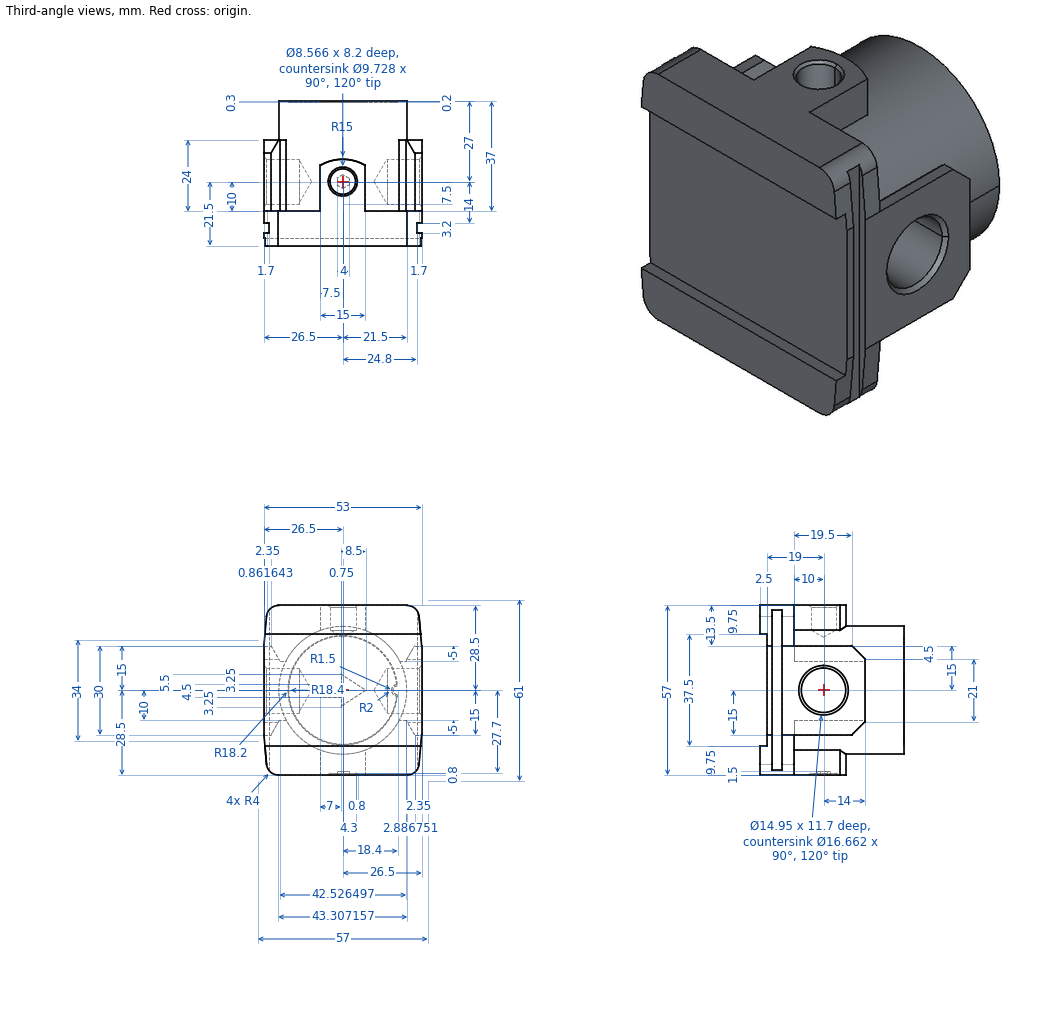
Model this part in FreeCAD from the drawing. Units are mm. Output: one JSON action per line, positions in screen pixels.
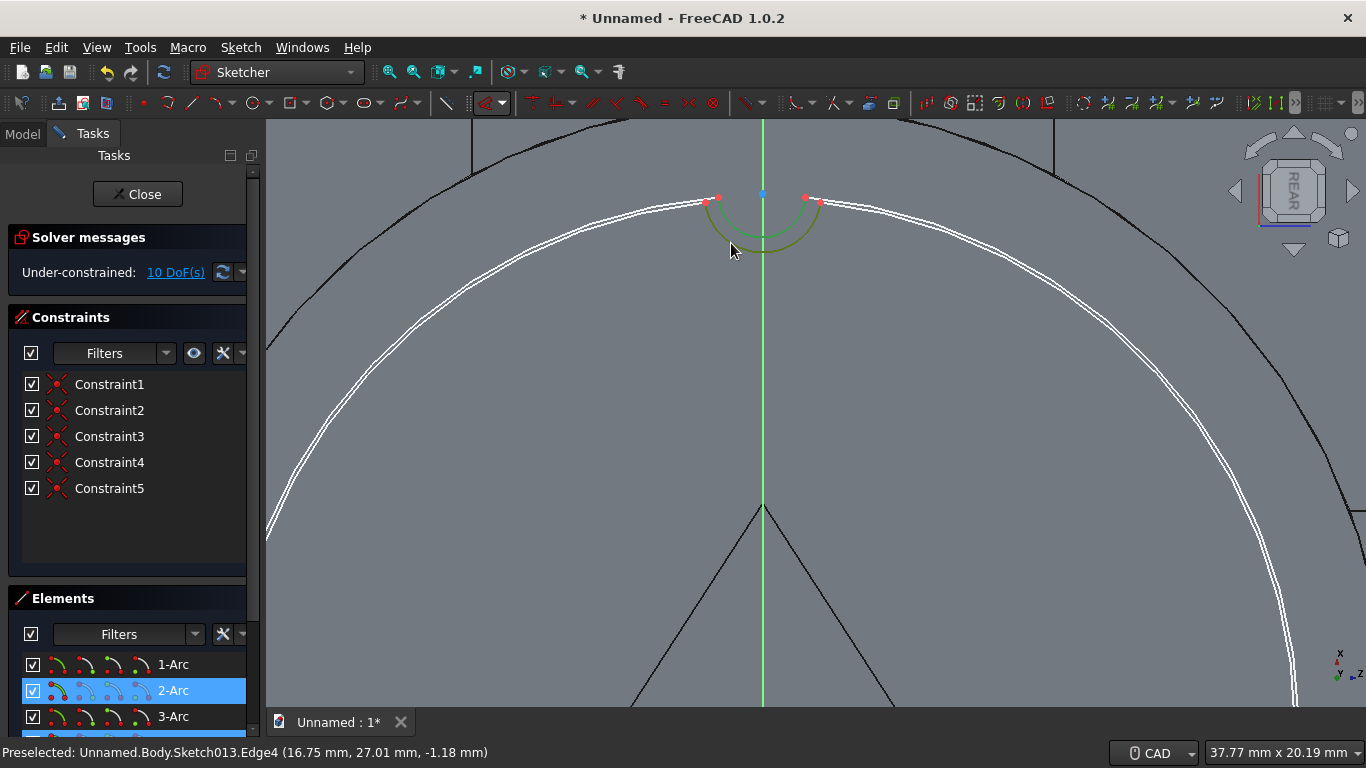
{"action": "left_click", "coordinate": [532, 104]}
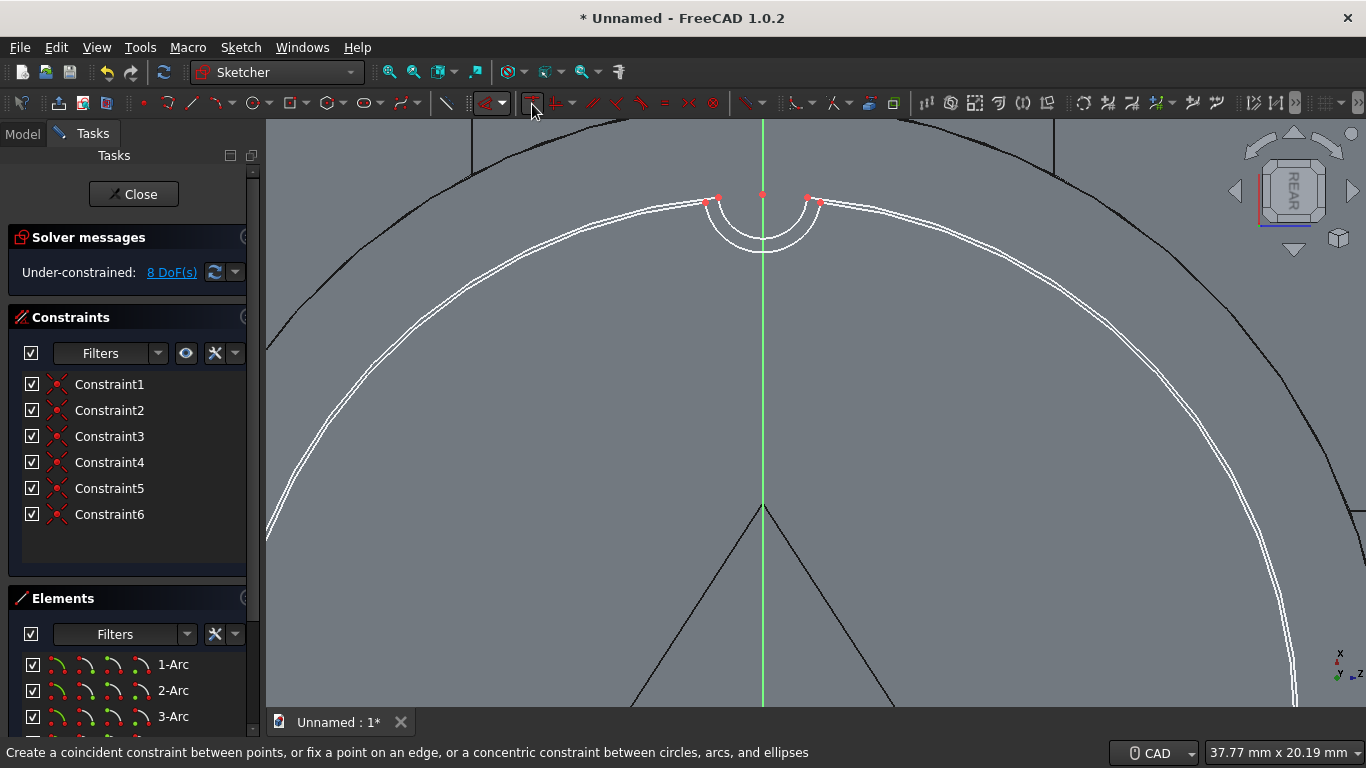
{"action": "scroll", "coordinate": [739, 229], "scroll_direction": "down", "scroll_amount": 5}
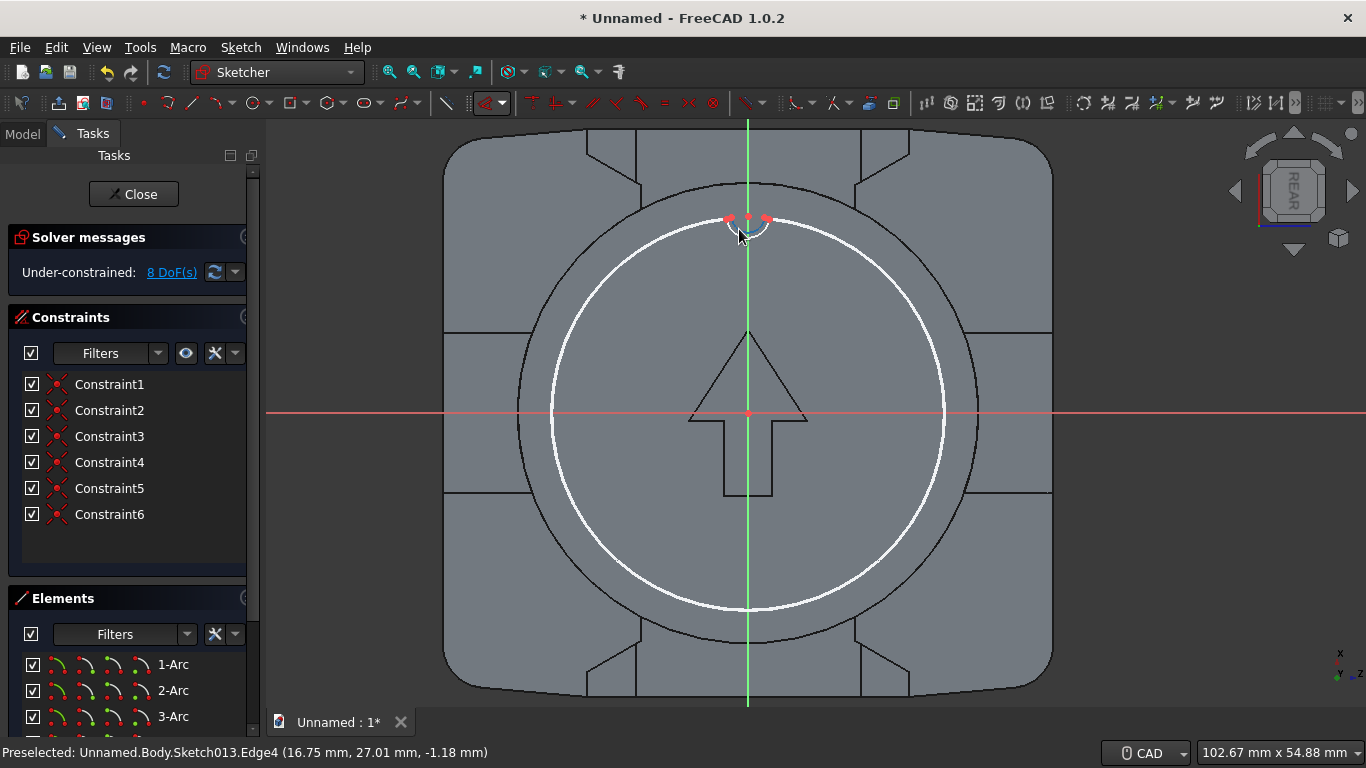
{"action": "scroll", "coordinate": [748, 414], "scroll_direction": "up", "scroll_amount": 5}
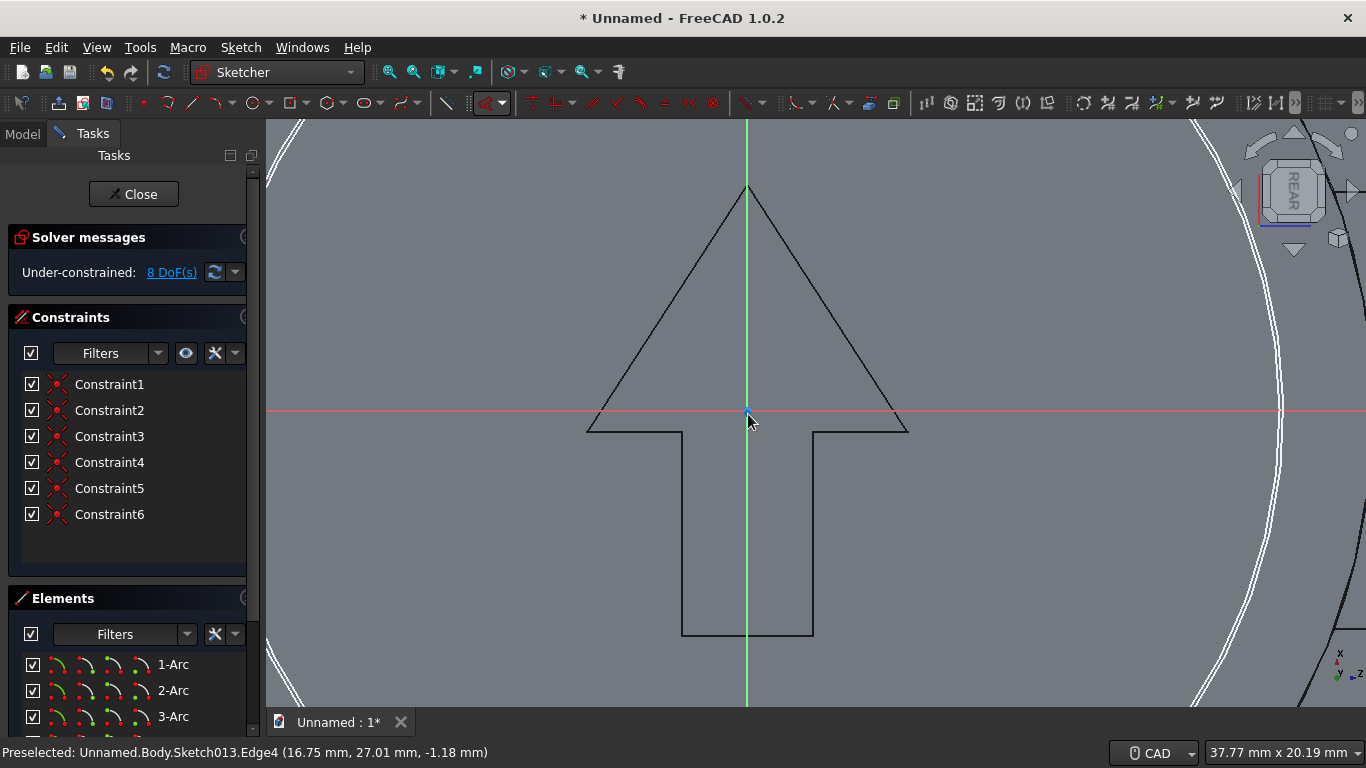
{"action": "left_click_drag", "start_coordinate": [737, 401], "coordinate": [757, 423]}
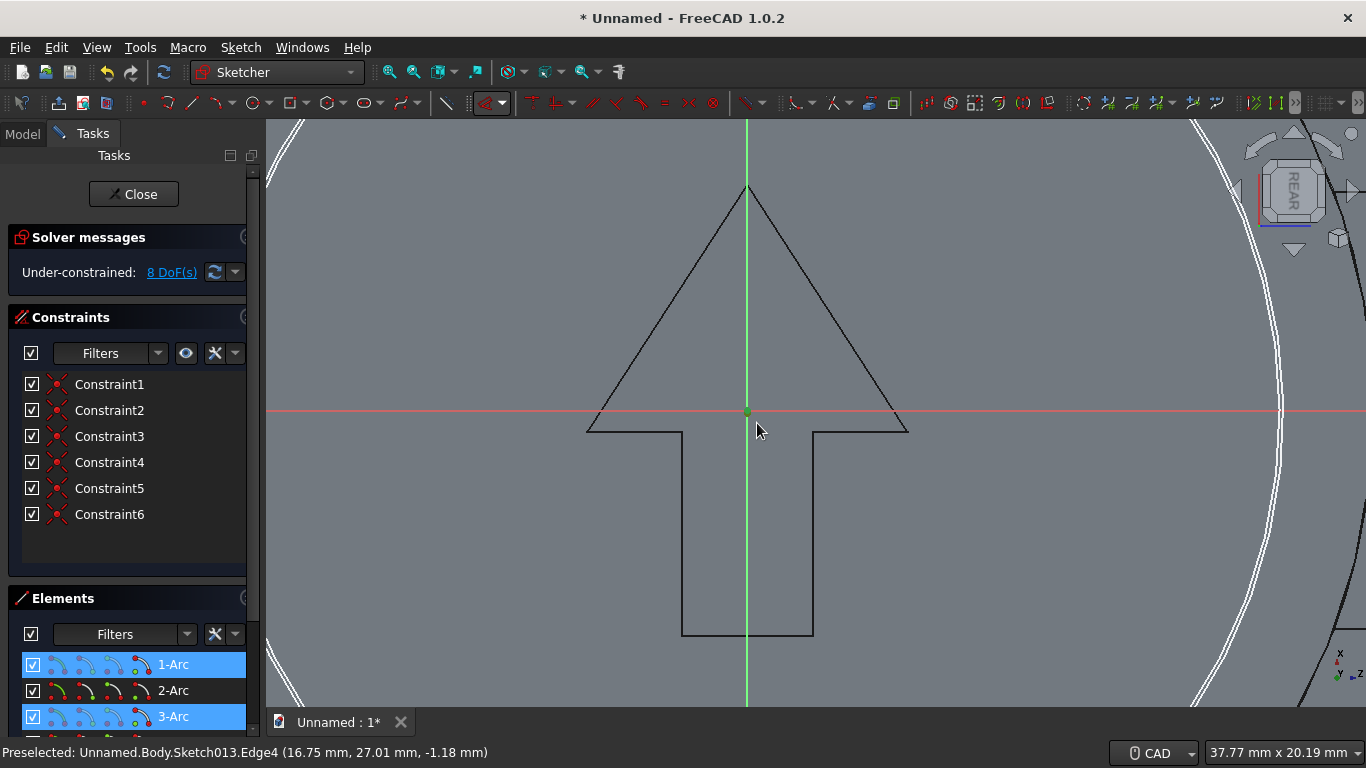
{"action": "left_click", "coordinate": [532, 104]}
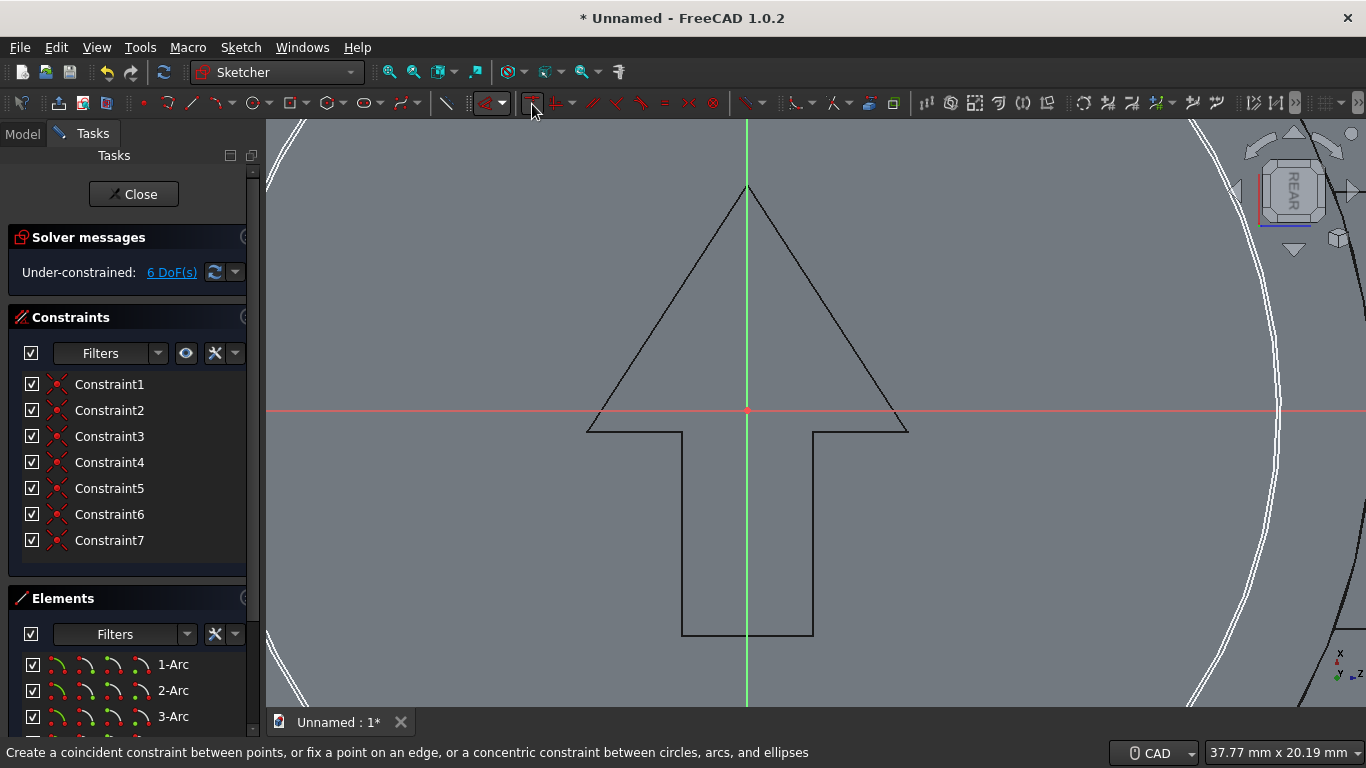
{"action": "scroll", "coordinate": [748, 414], "scroll_direction": "down", "scroll_amount": 5}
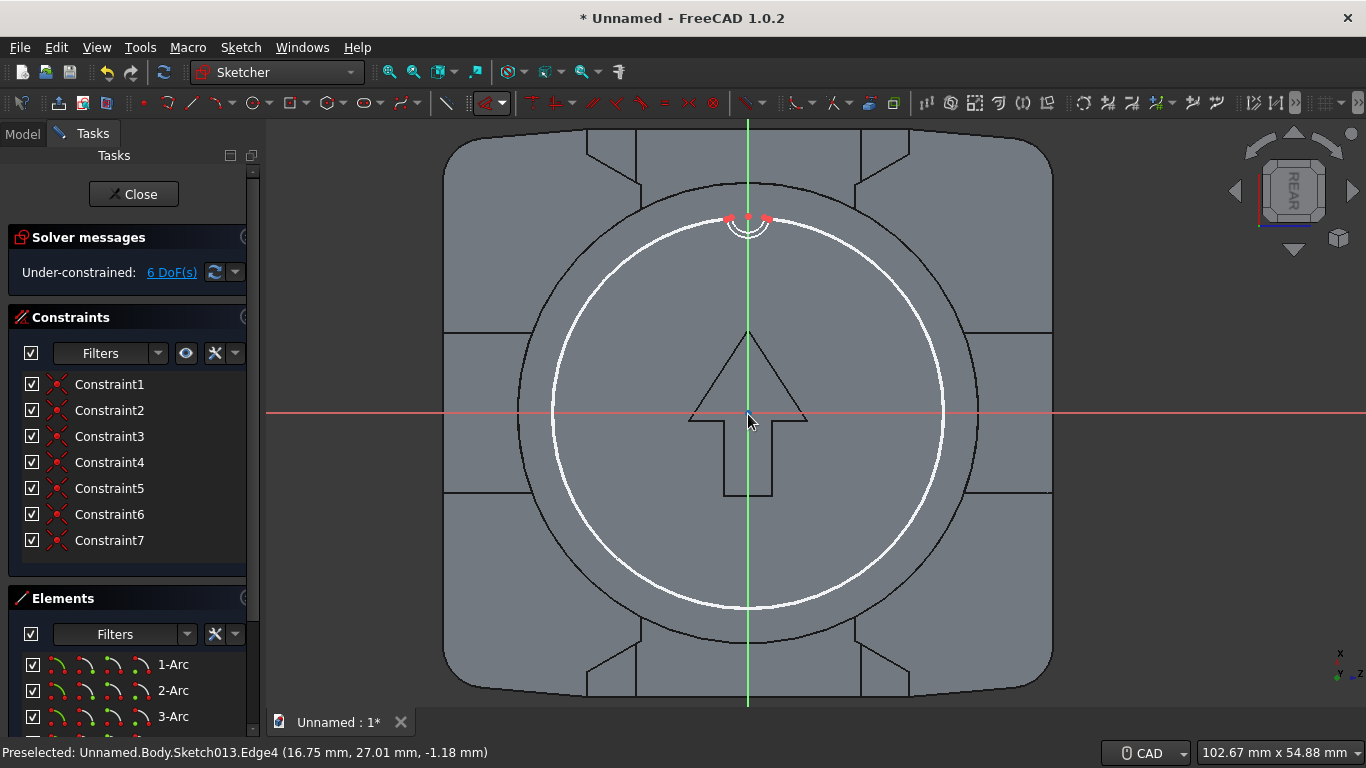
{"action": "left_click", "coordinate": [748, 216]}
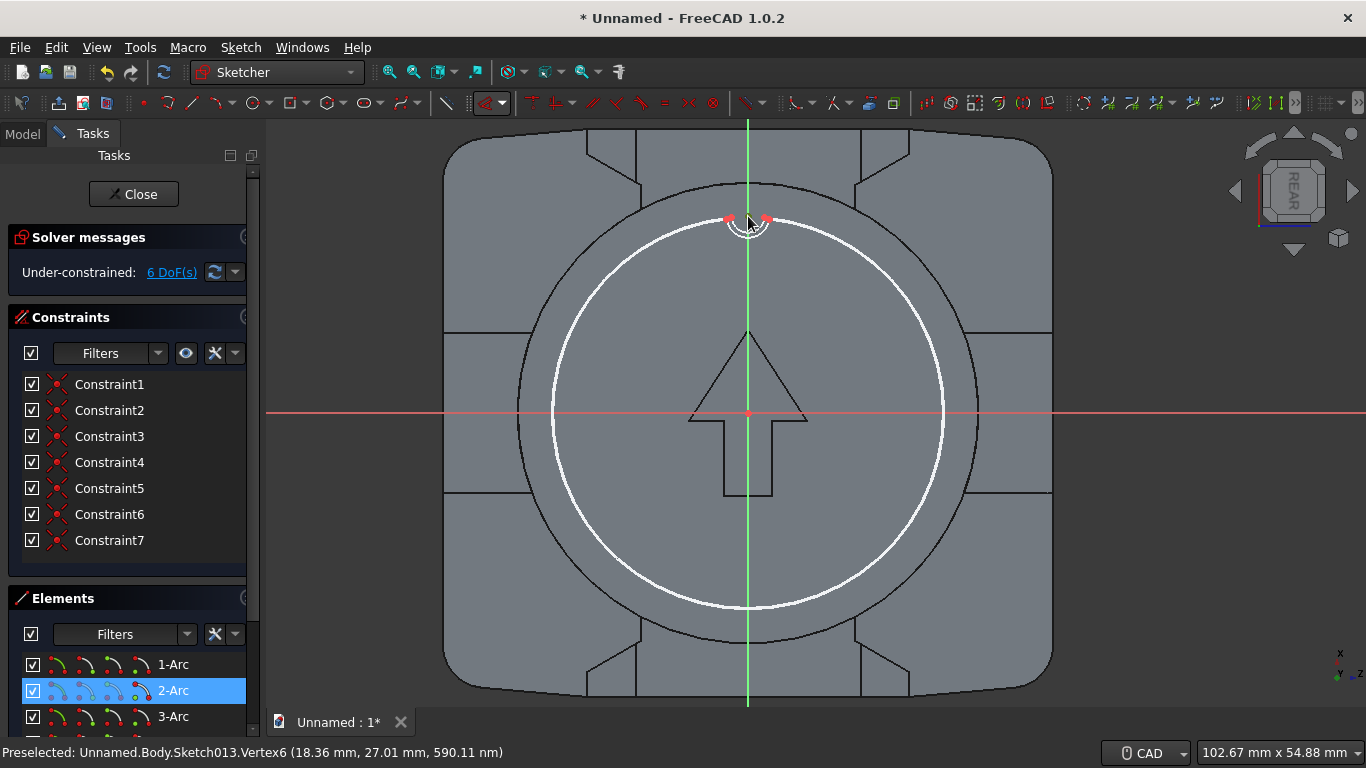
{"action": "left_click", "coordinate": [748, 641]}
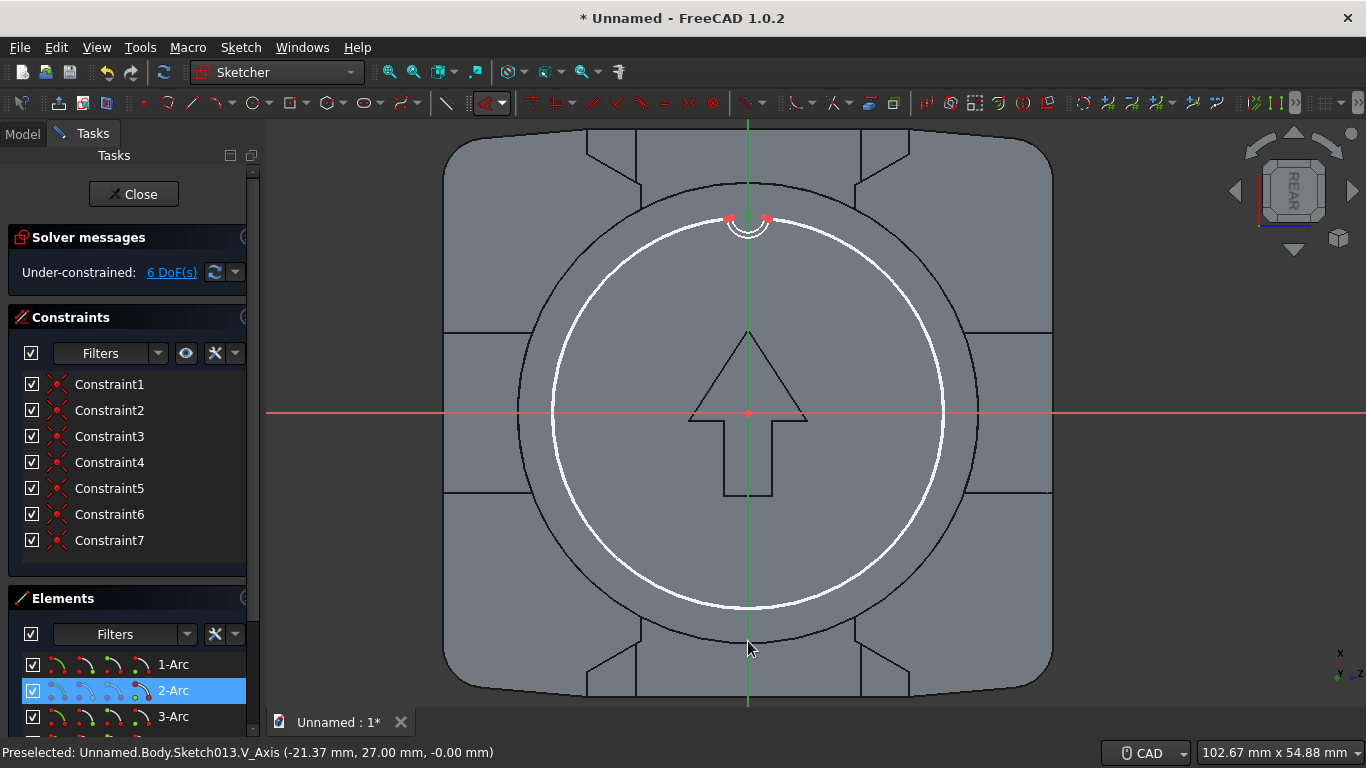
{"action": "left_click", "coordinate": [532, 104]}